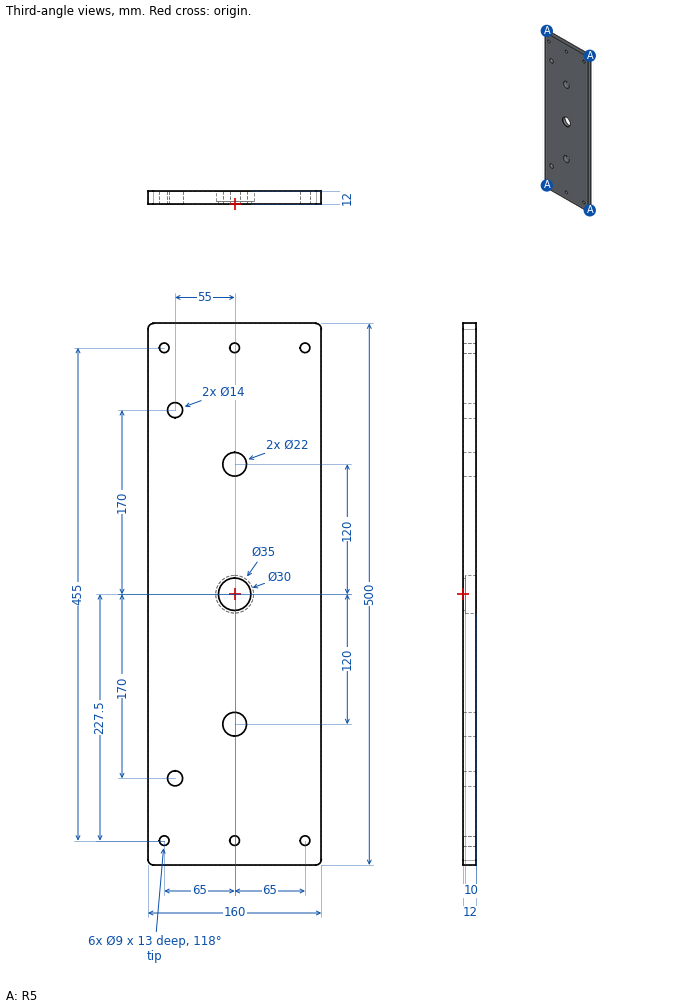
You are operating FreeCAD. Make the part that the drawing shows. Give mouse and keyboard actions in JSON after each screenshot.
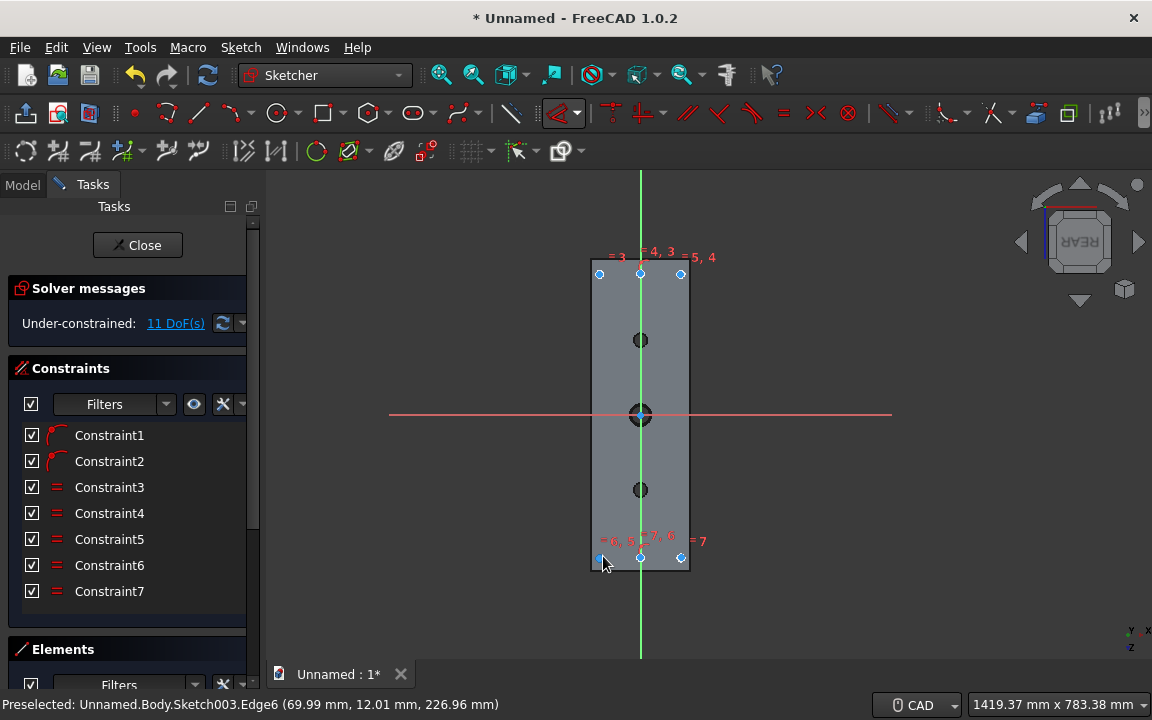
{"action": "scroll", "coordinate": [602, 272], "scroll_direction": "up", "scroll_amount": 10}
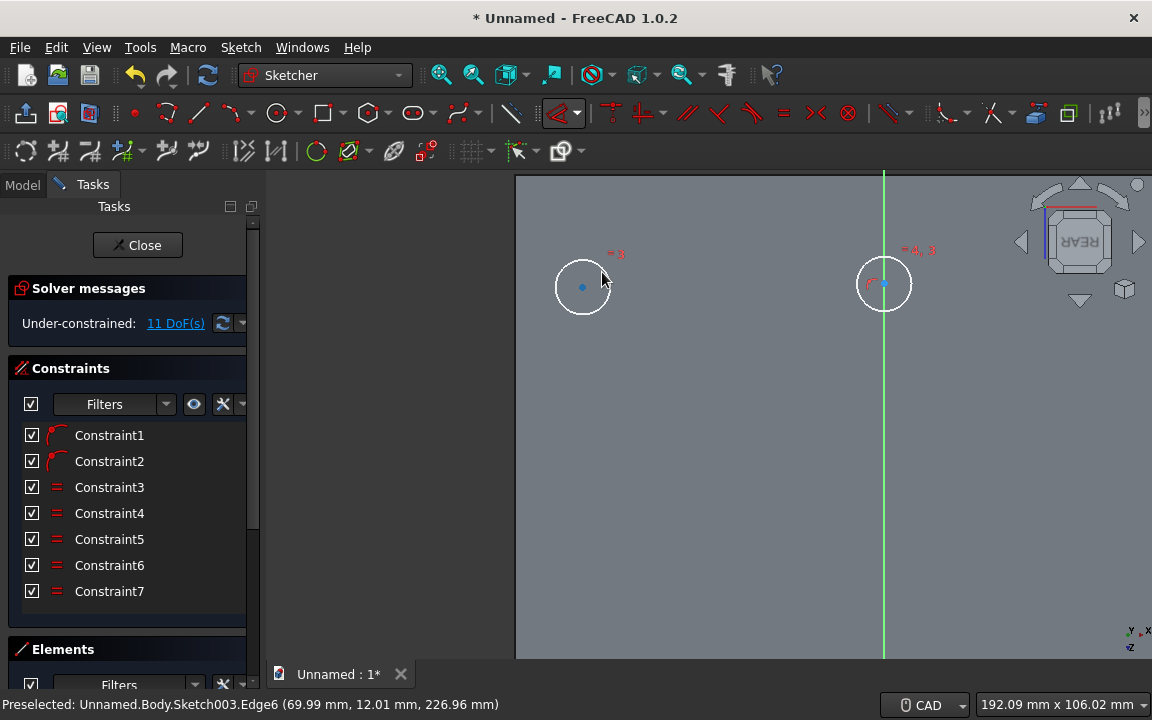
{"action": "left_click", "coordinate": [602, 268]}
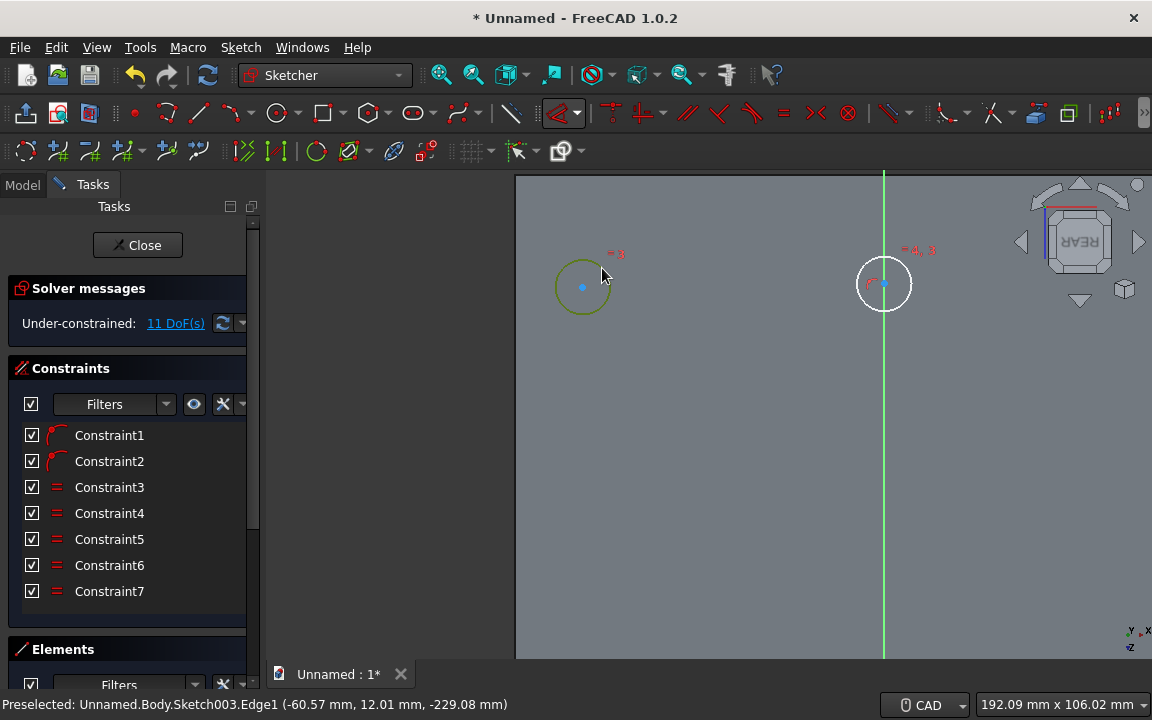
{"action": "left_click", "coordinate": [580, 114]}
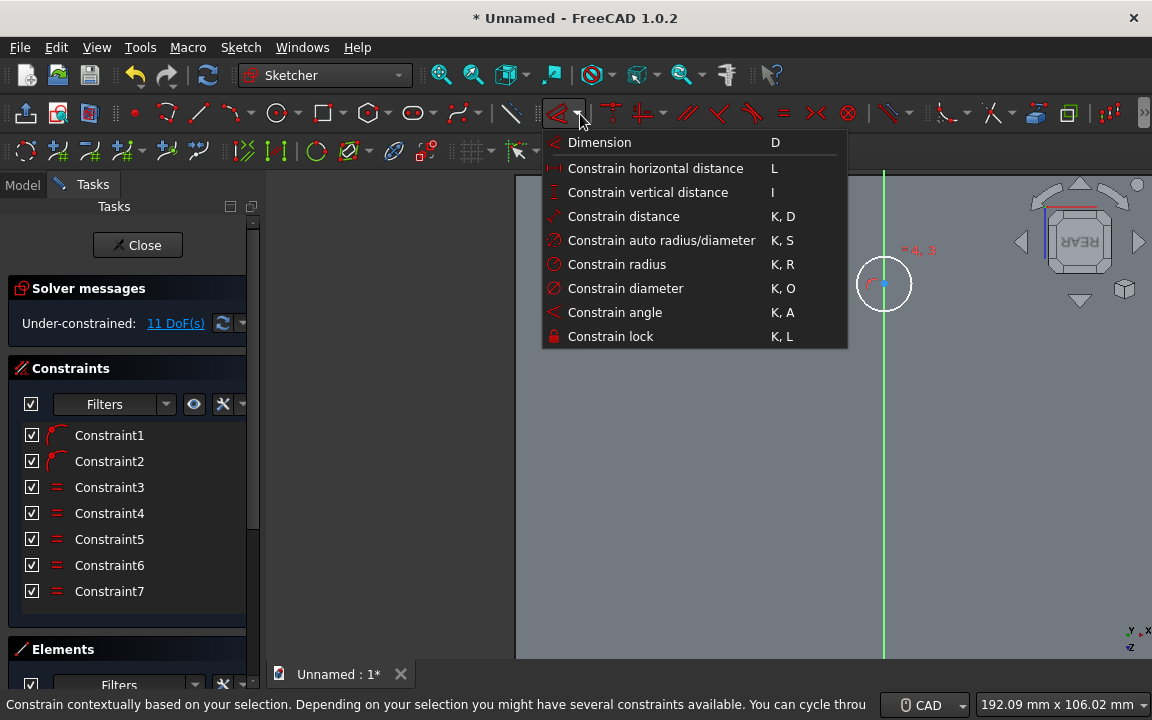
{"action": "left_click", "coordinate": [695, 288]}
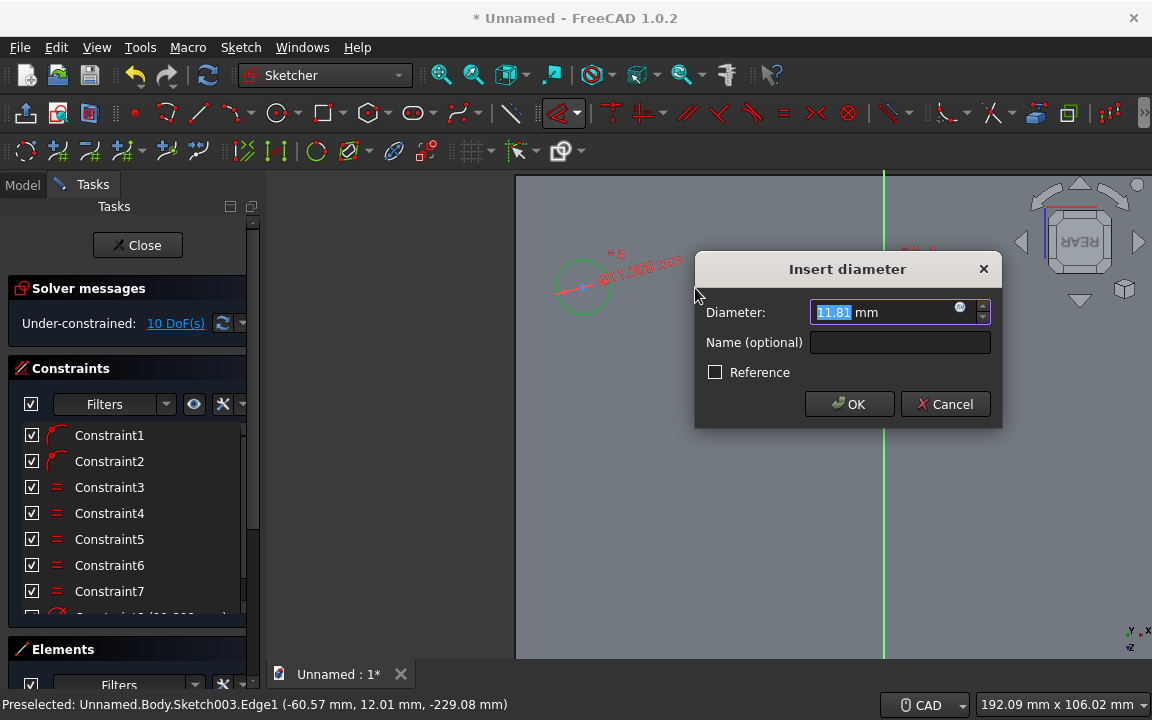
{"action": "type", "text": "9"}
{"action": "key", "text": "Return"}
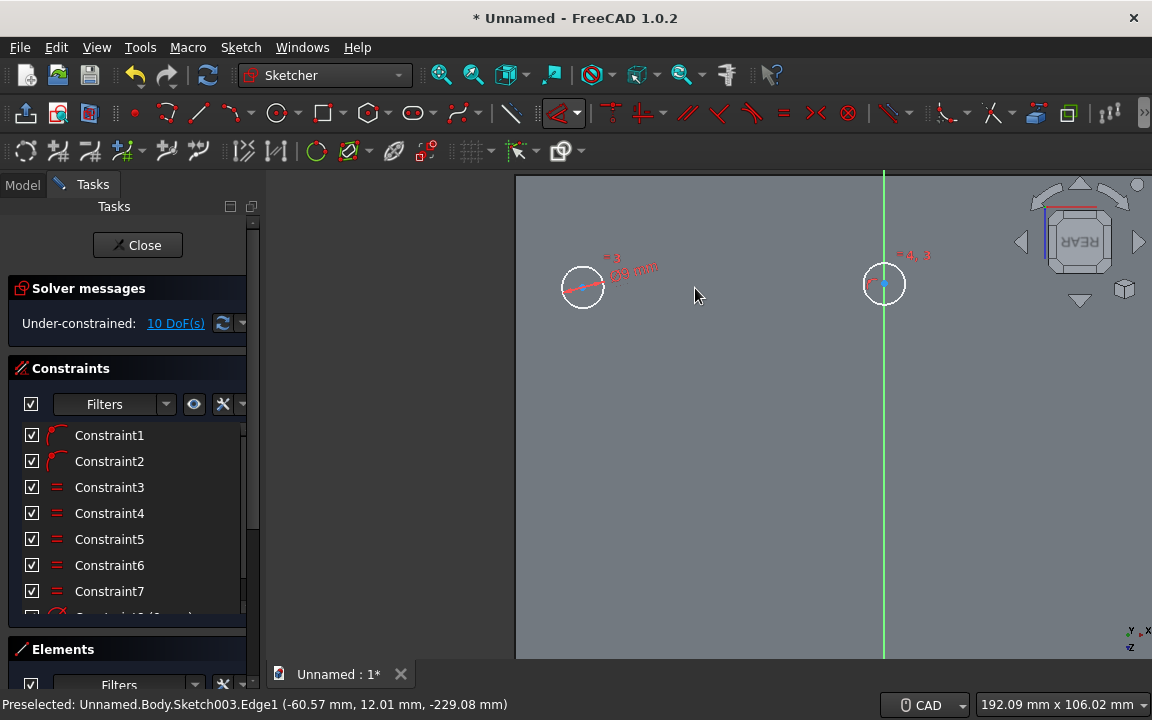
{"action": "scroll", "coordinate": [602, 272], "scroll_direction": "down", "scroll_amount": 10}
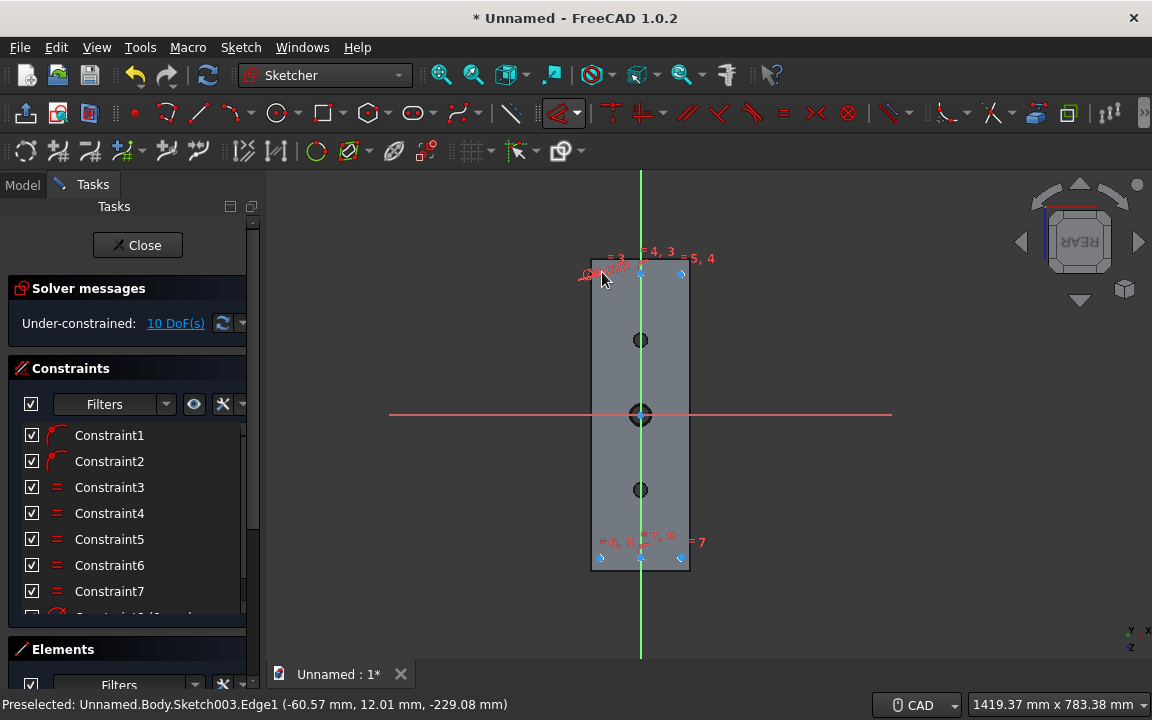
{"action": "left_click", "coordinate": [600, 274]}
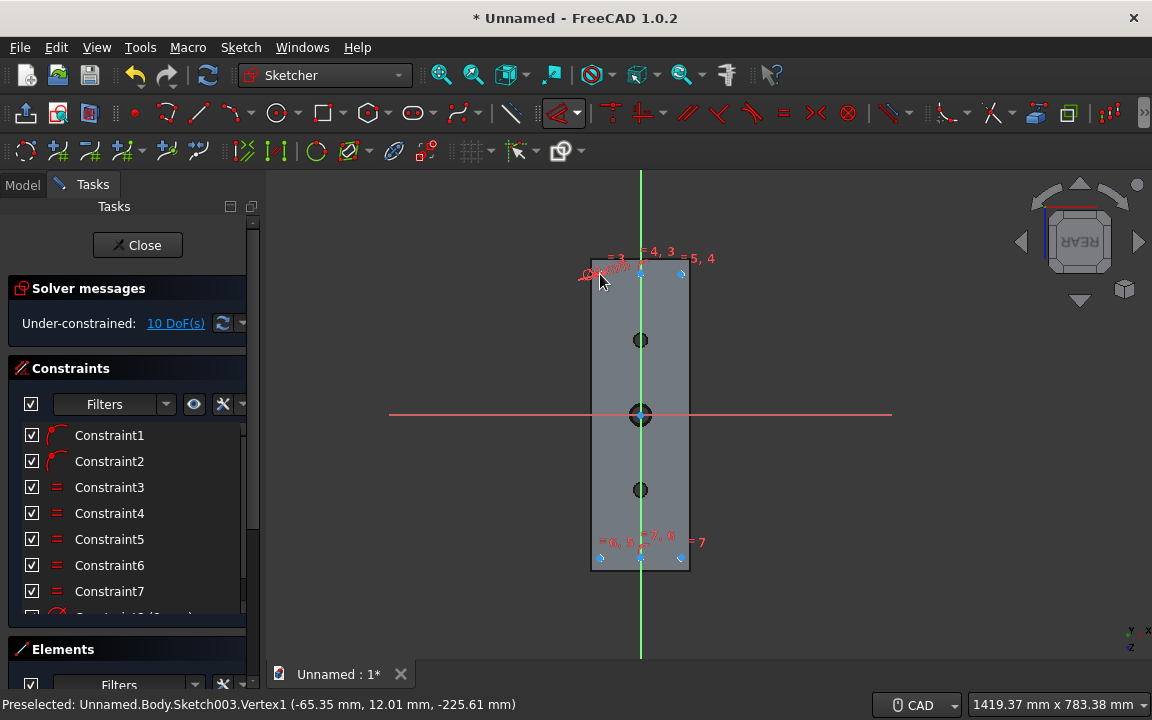
{"action": "key", "text": "l"}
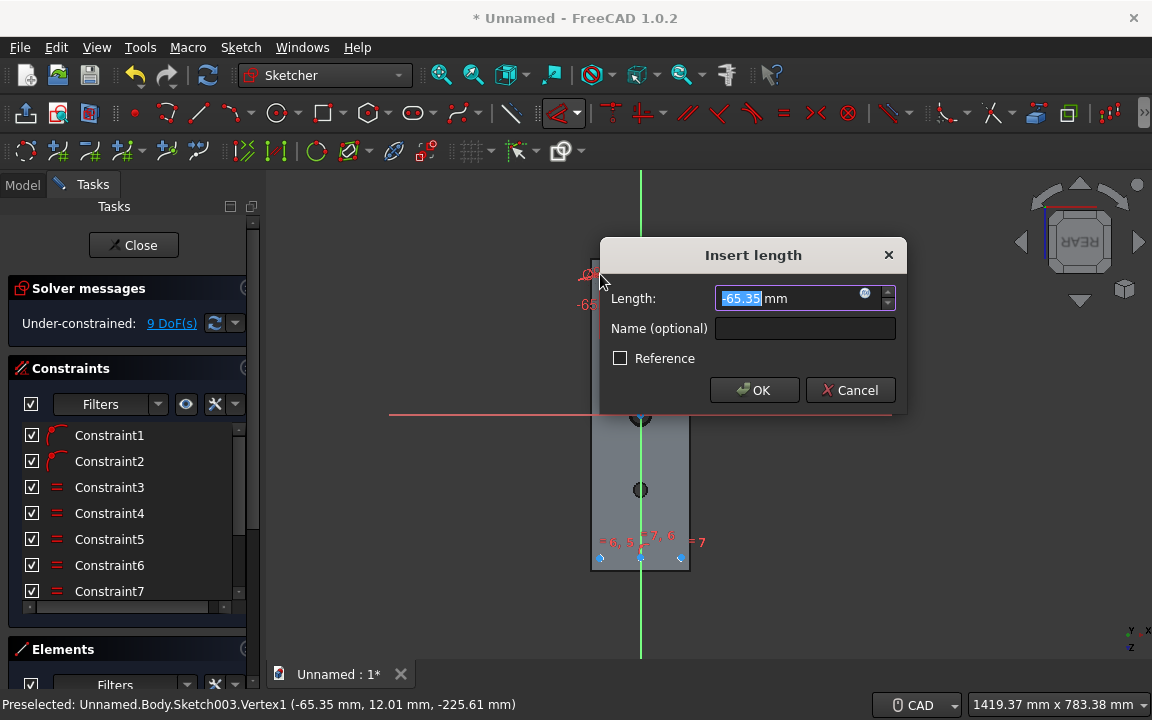
{"action": "type", "text": "-65"}
{"action": "key", "text": "Return"}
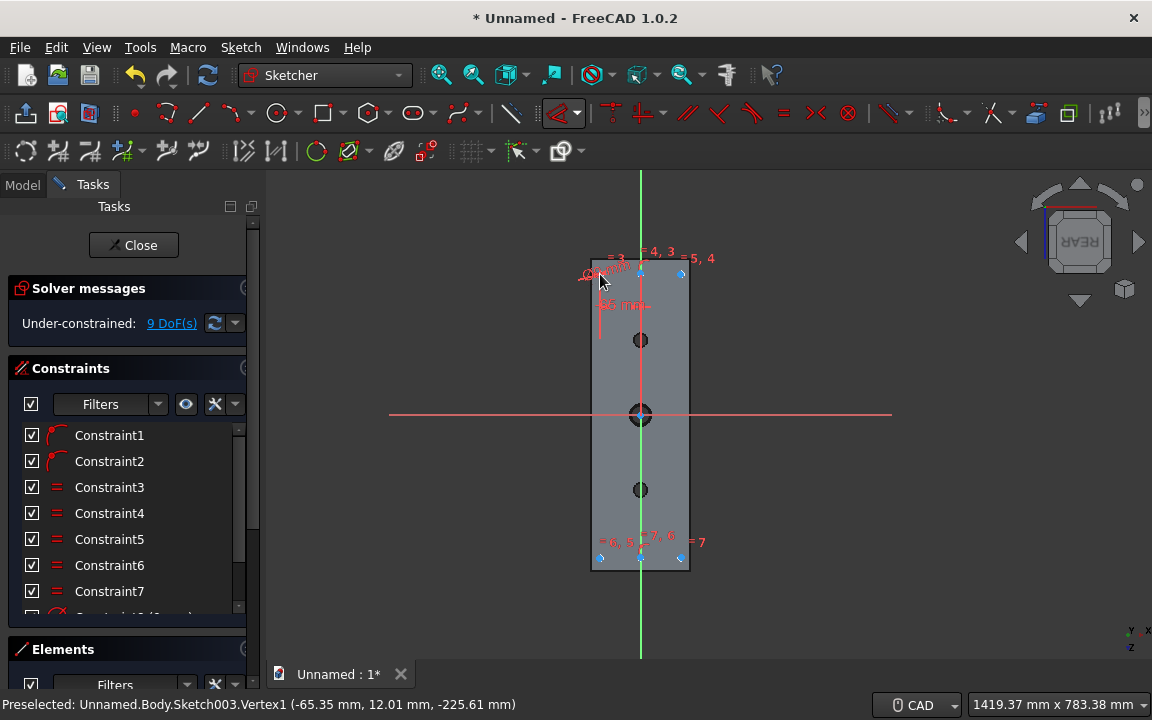
{"action": "left_click", "coordinate": [681, 274]}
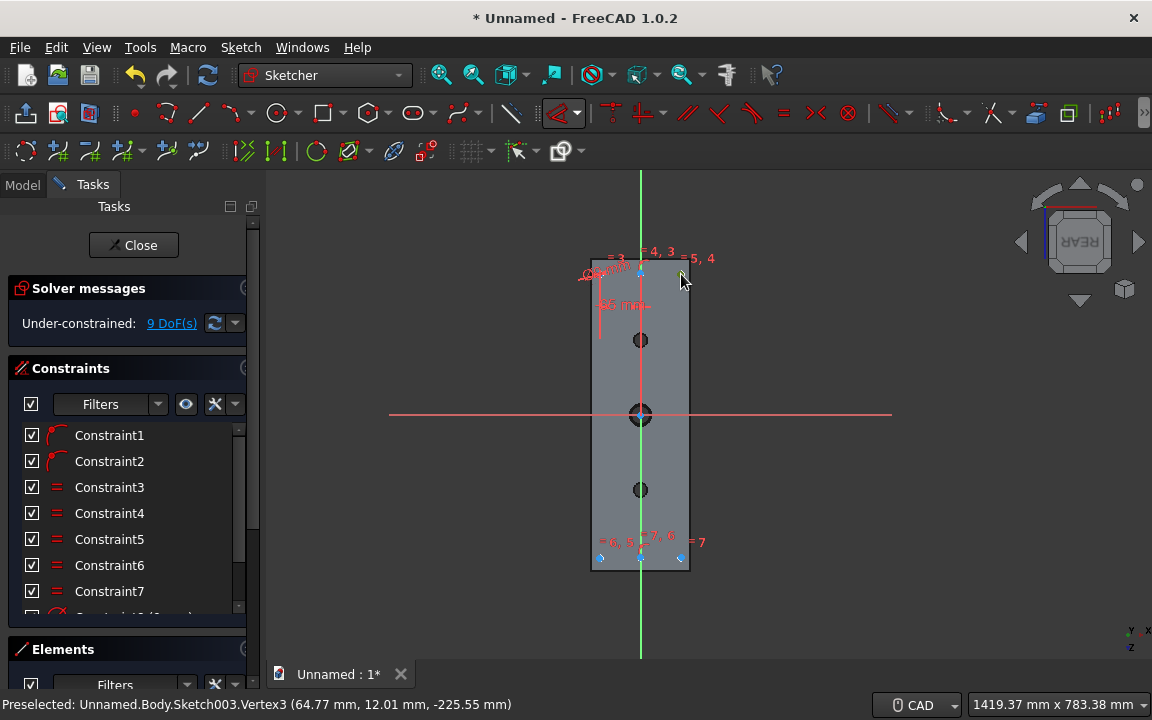
{"action": "left_click", "coordinate": [580, 114]}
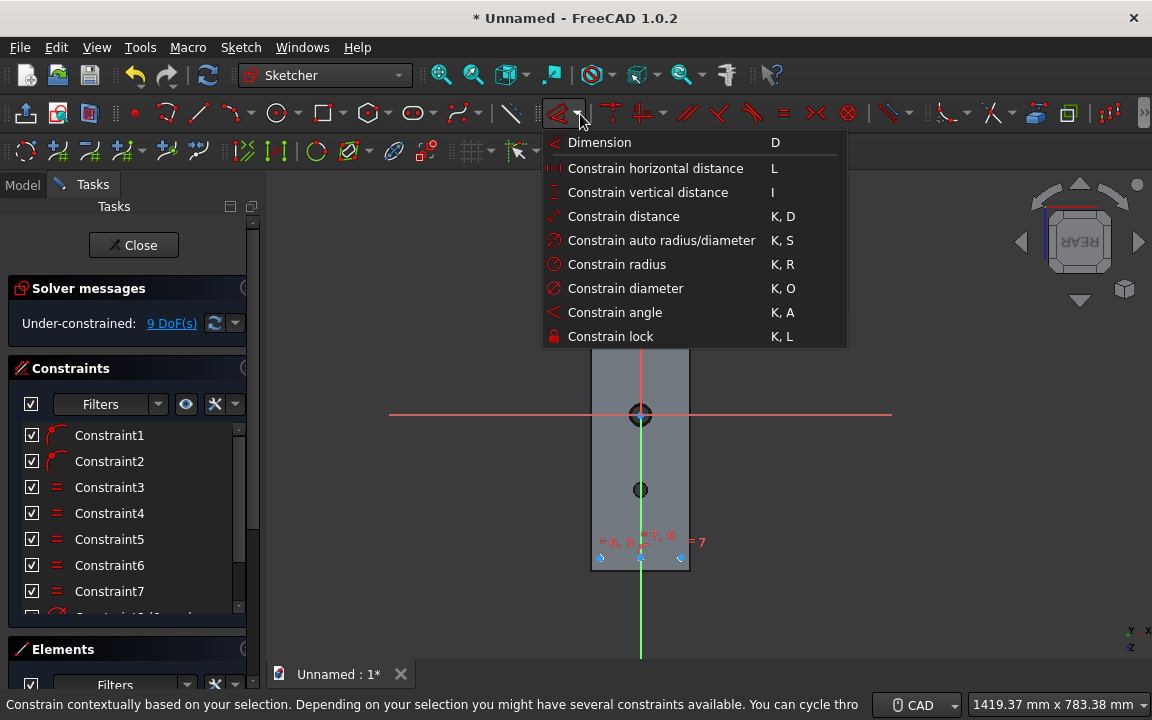
{"action": "left_click", "coordinate": [695, 168]}